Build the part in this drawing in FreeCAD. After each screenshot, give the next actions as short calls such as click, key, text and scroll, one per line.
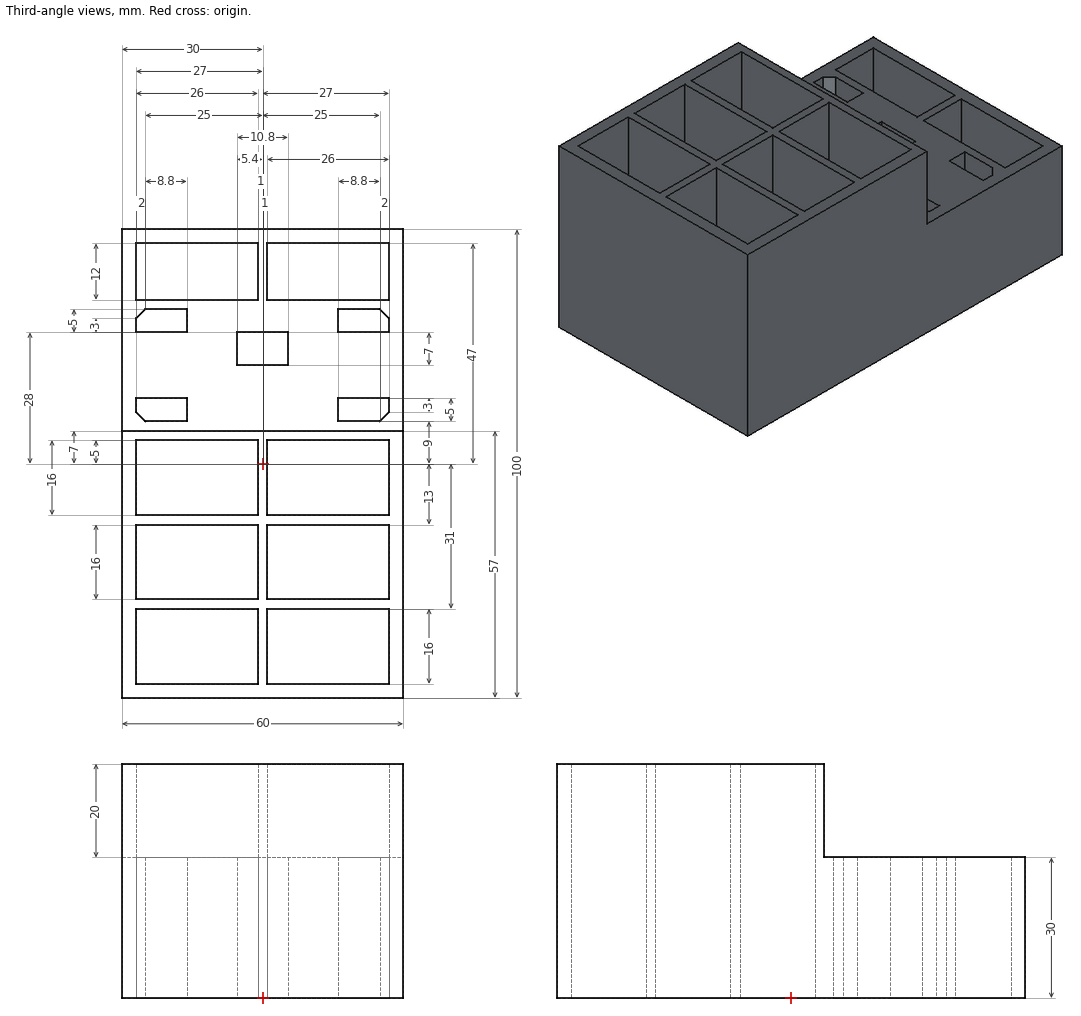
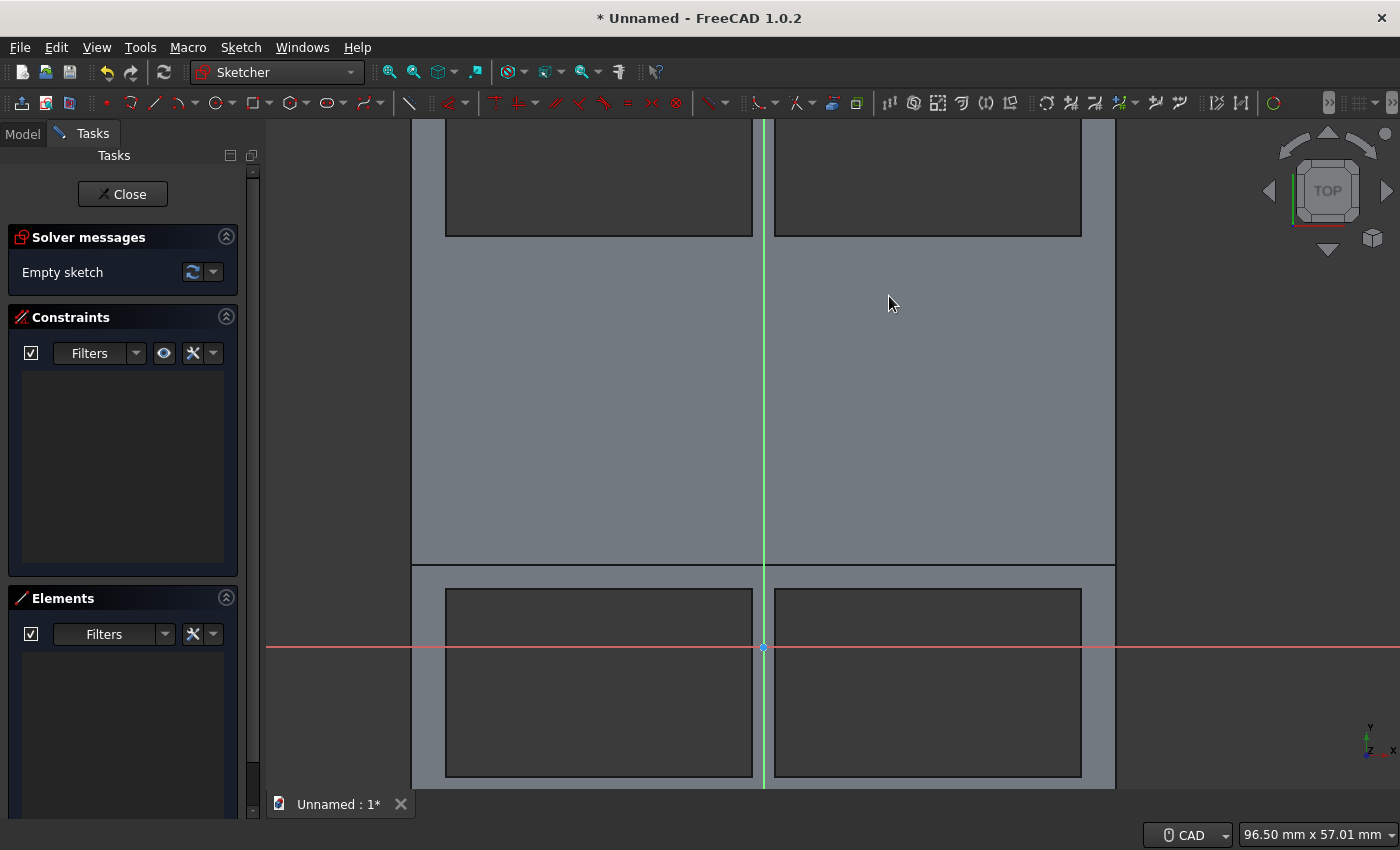
click(132, 104)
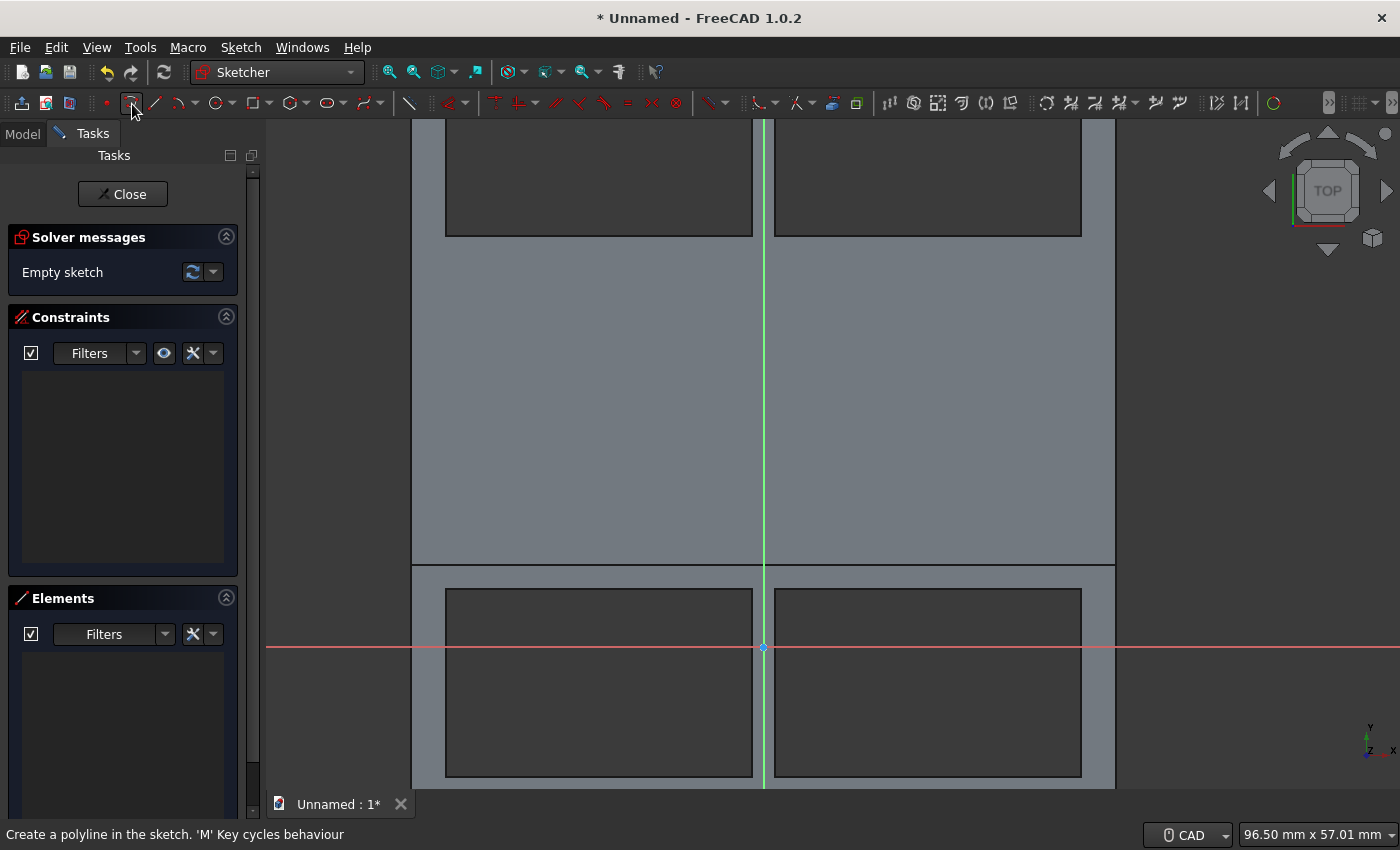
click(954, 542)
click(1057, 542)
click(1081, 518)
click(1081, 483)
click(954, 483)
click(954, 543)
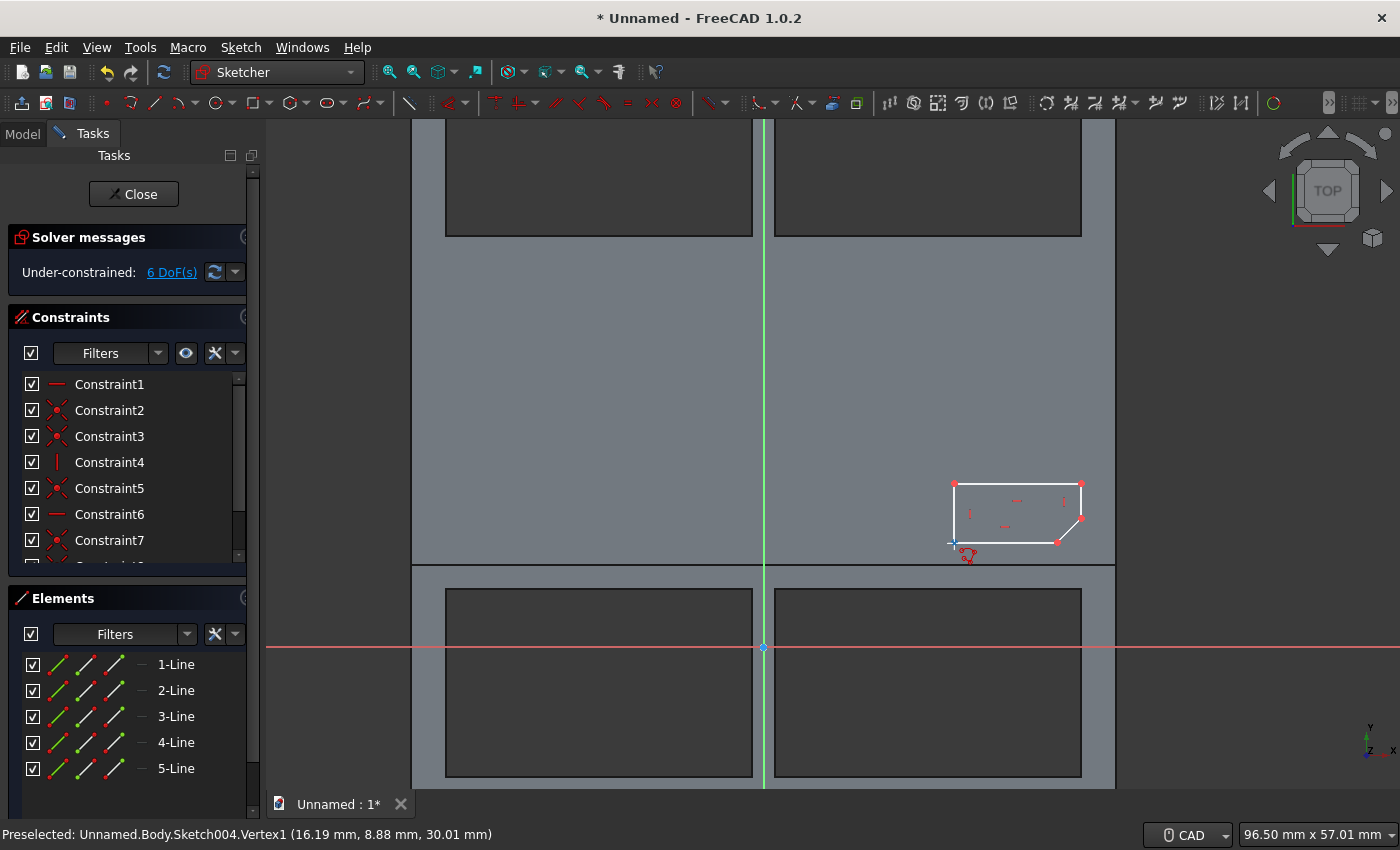
key(g)
key(r)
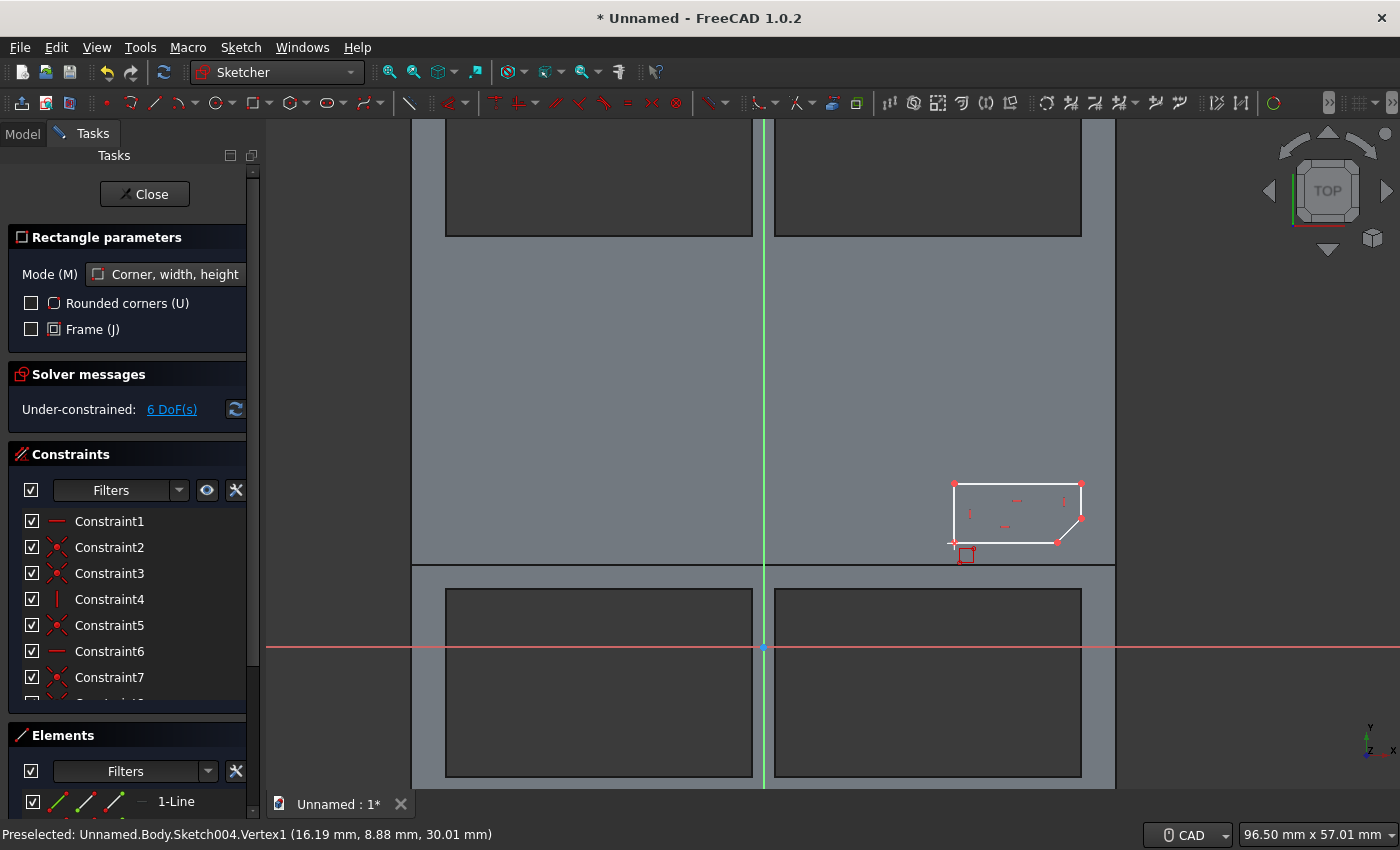
click(700, 318)
move(827, 401)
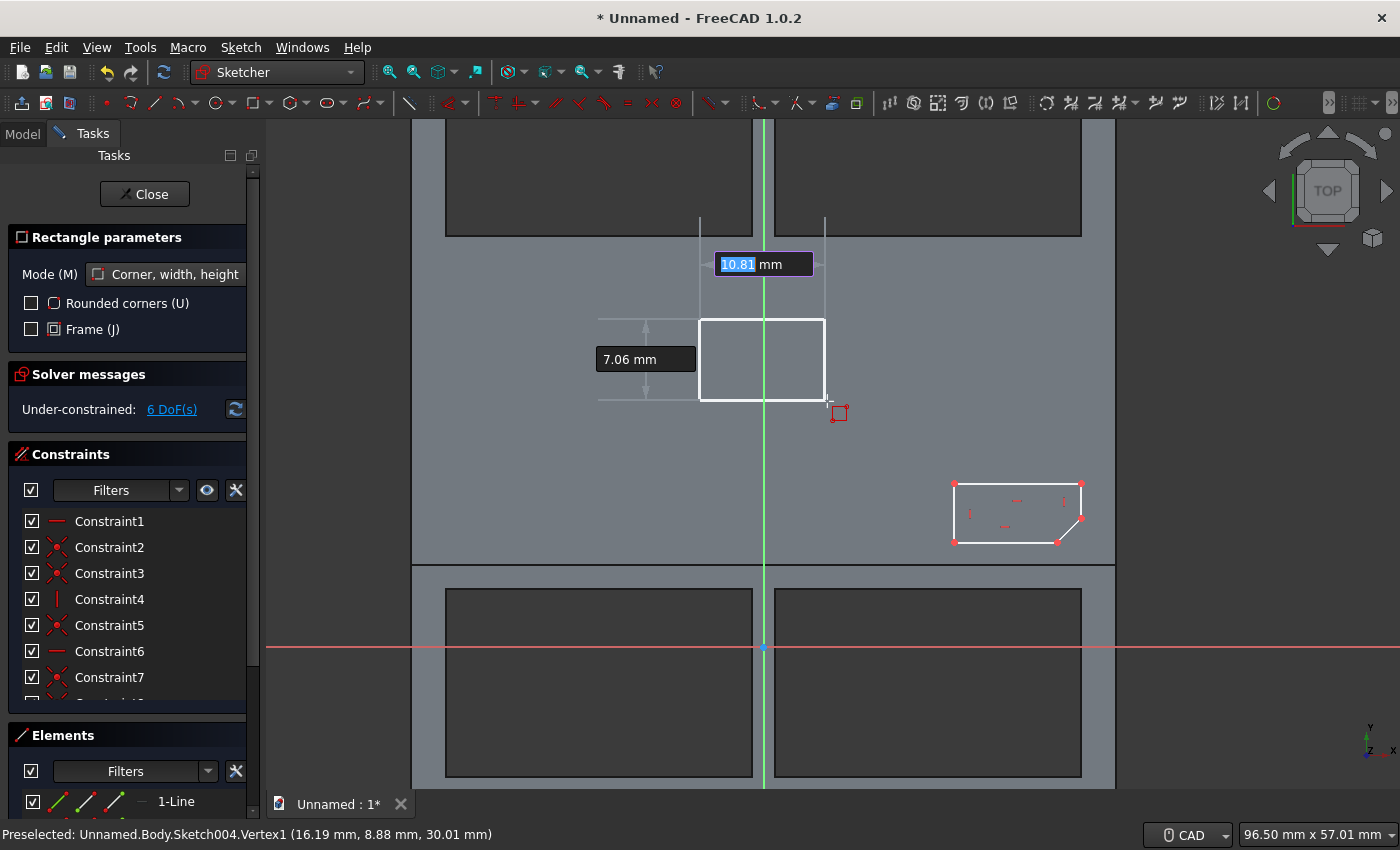
text(10.8)
key(Tab)
text(7)
key(Return)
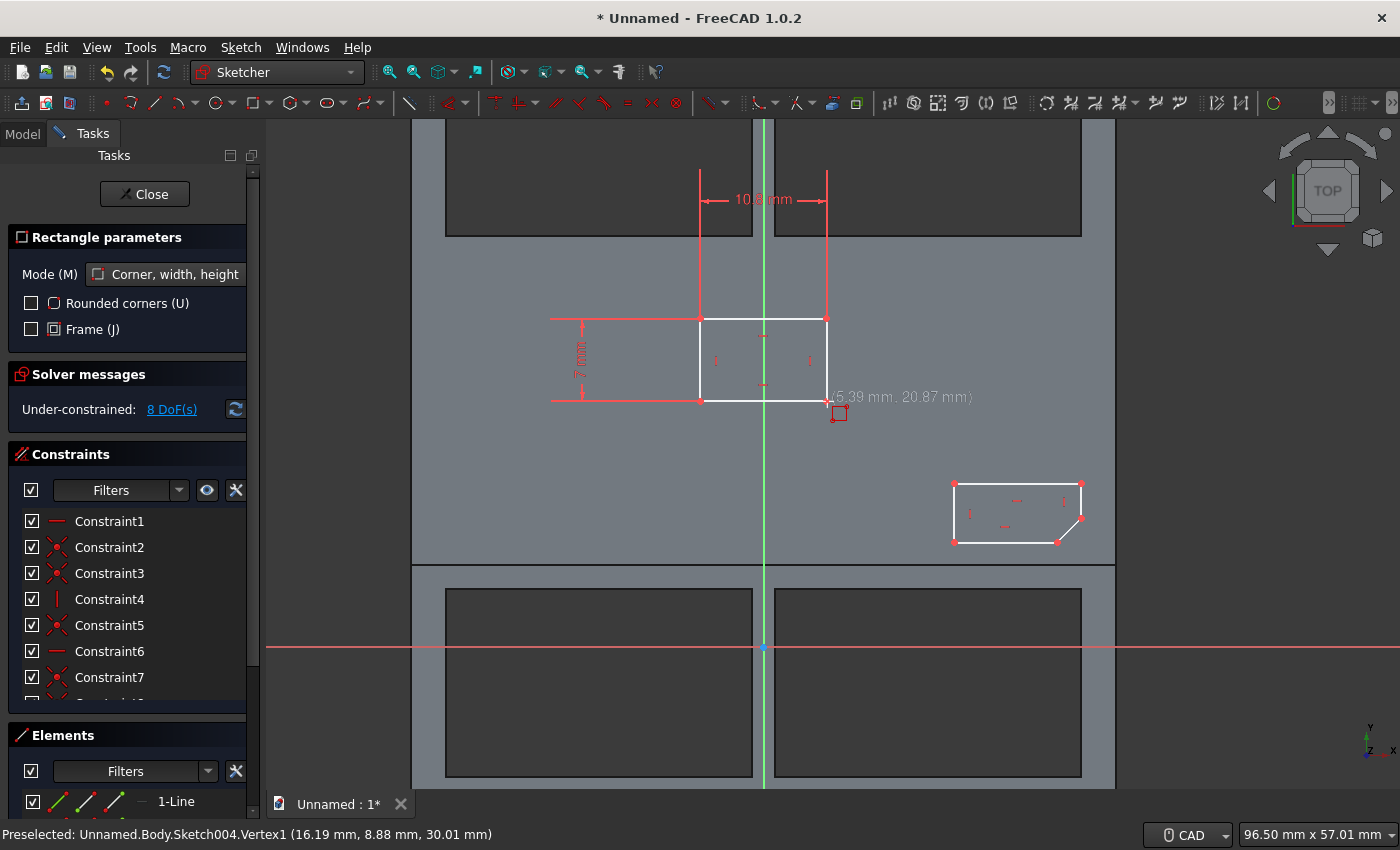
key(g)
key(m)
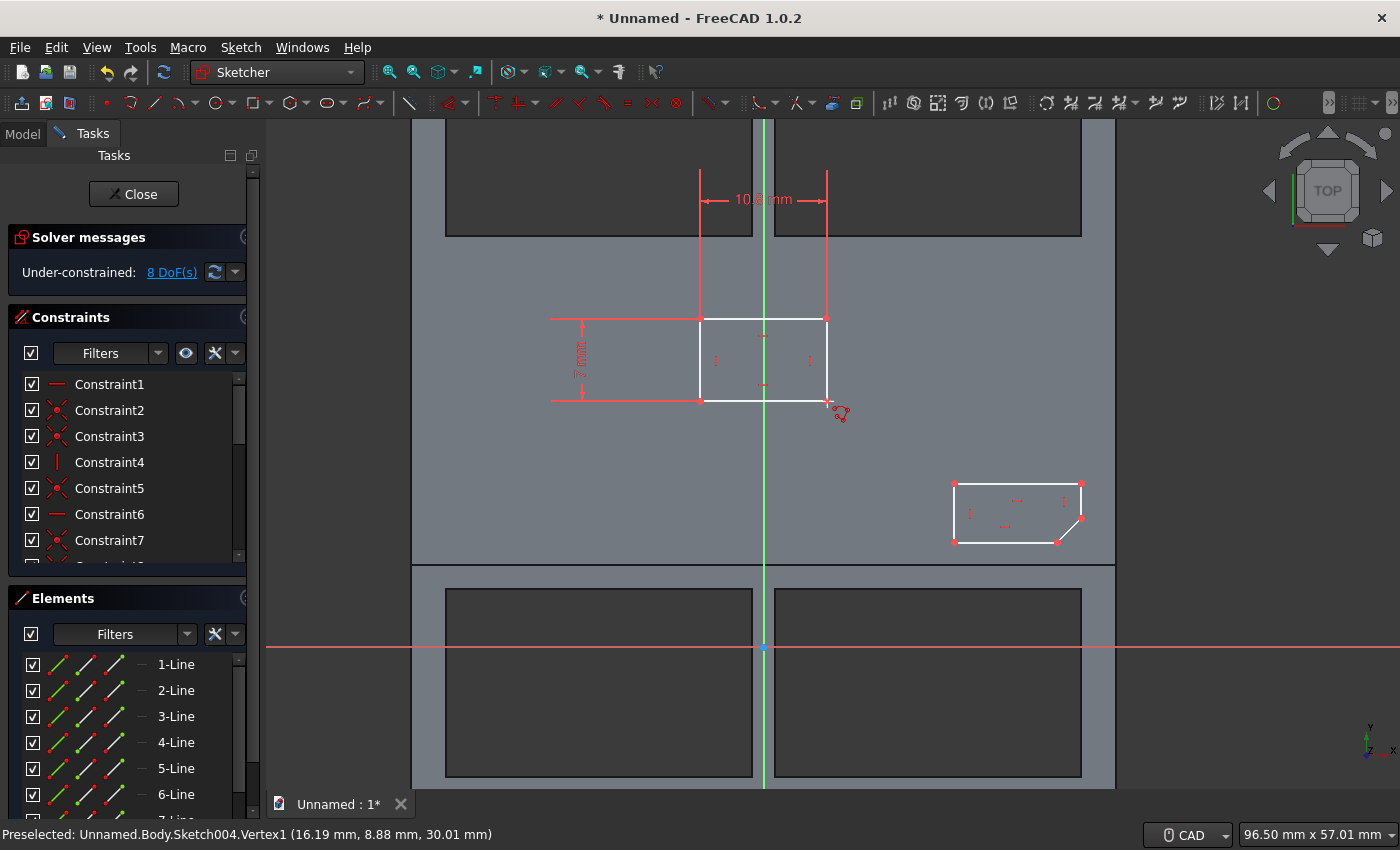
click(573, 318)
click(573, 260)
click(470, 260)
click(446, 283)
click(446, 318)
click(573, 319)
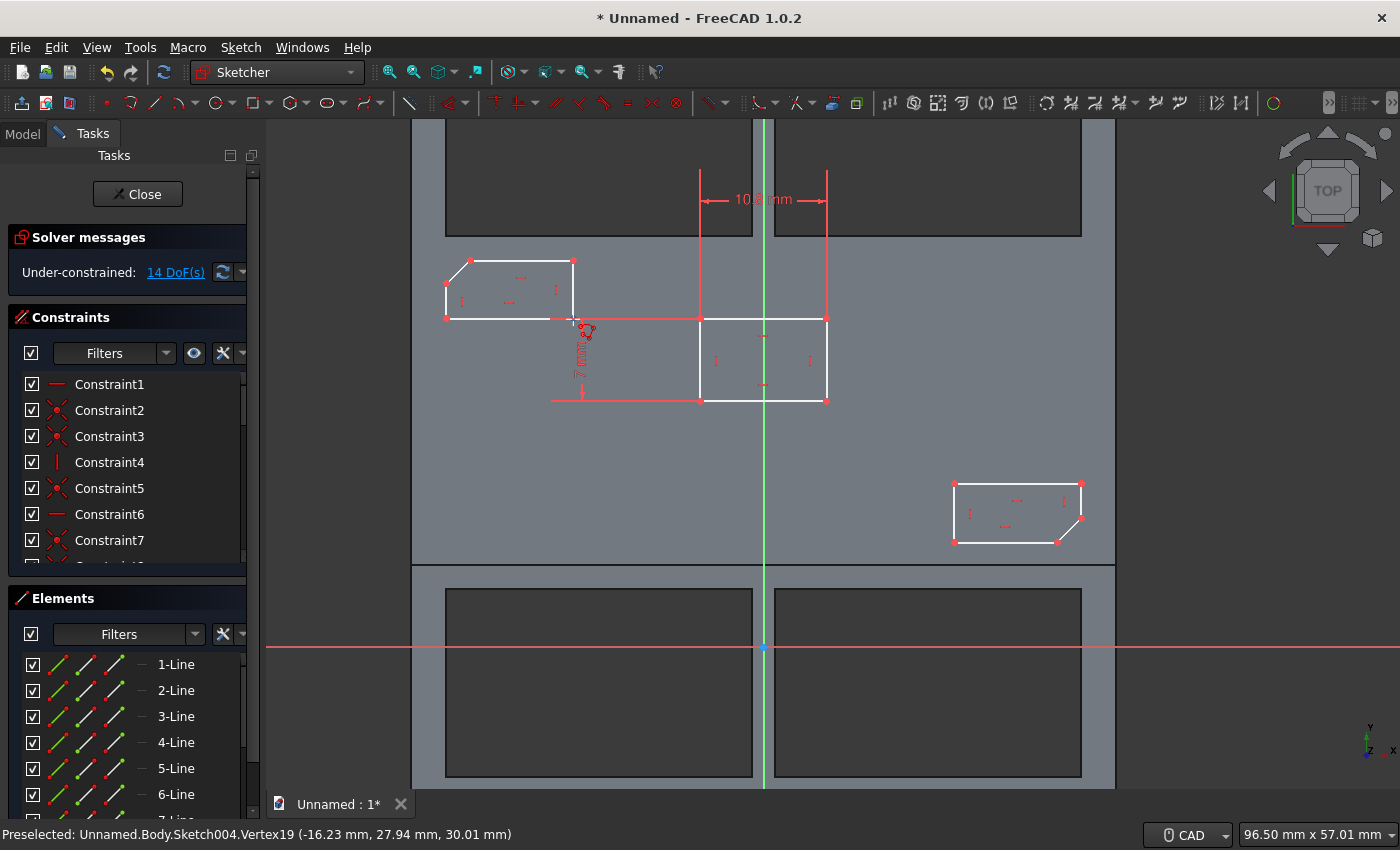
click(954, 318)
click(1081, 318)
click(1081, 283)
click(1057, 260)
click(954, 260)
click(954, 319)